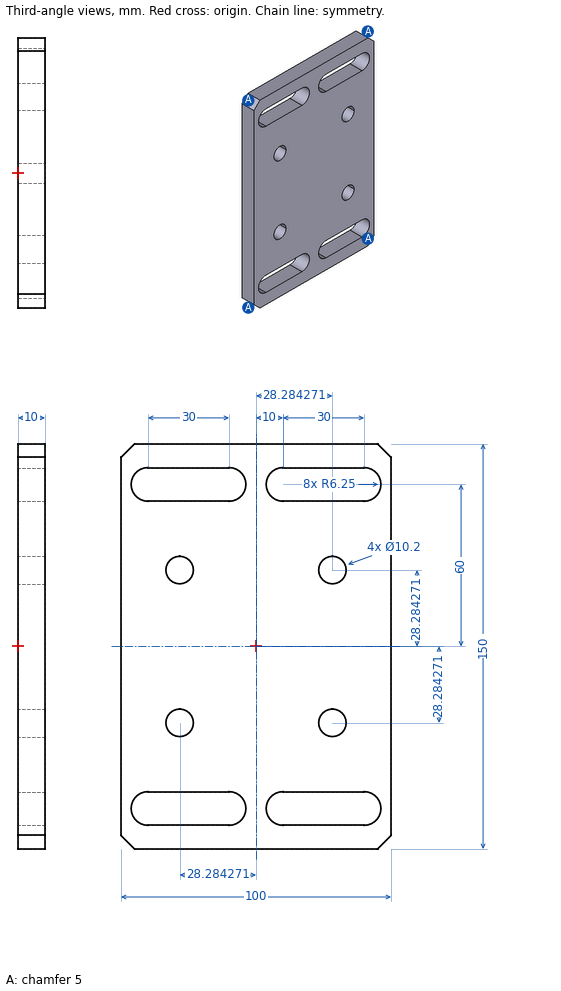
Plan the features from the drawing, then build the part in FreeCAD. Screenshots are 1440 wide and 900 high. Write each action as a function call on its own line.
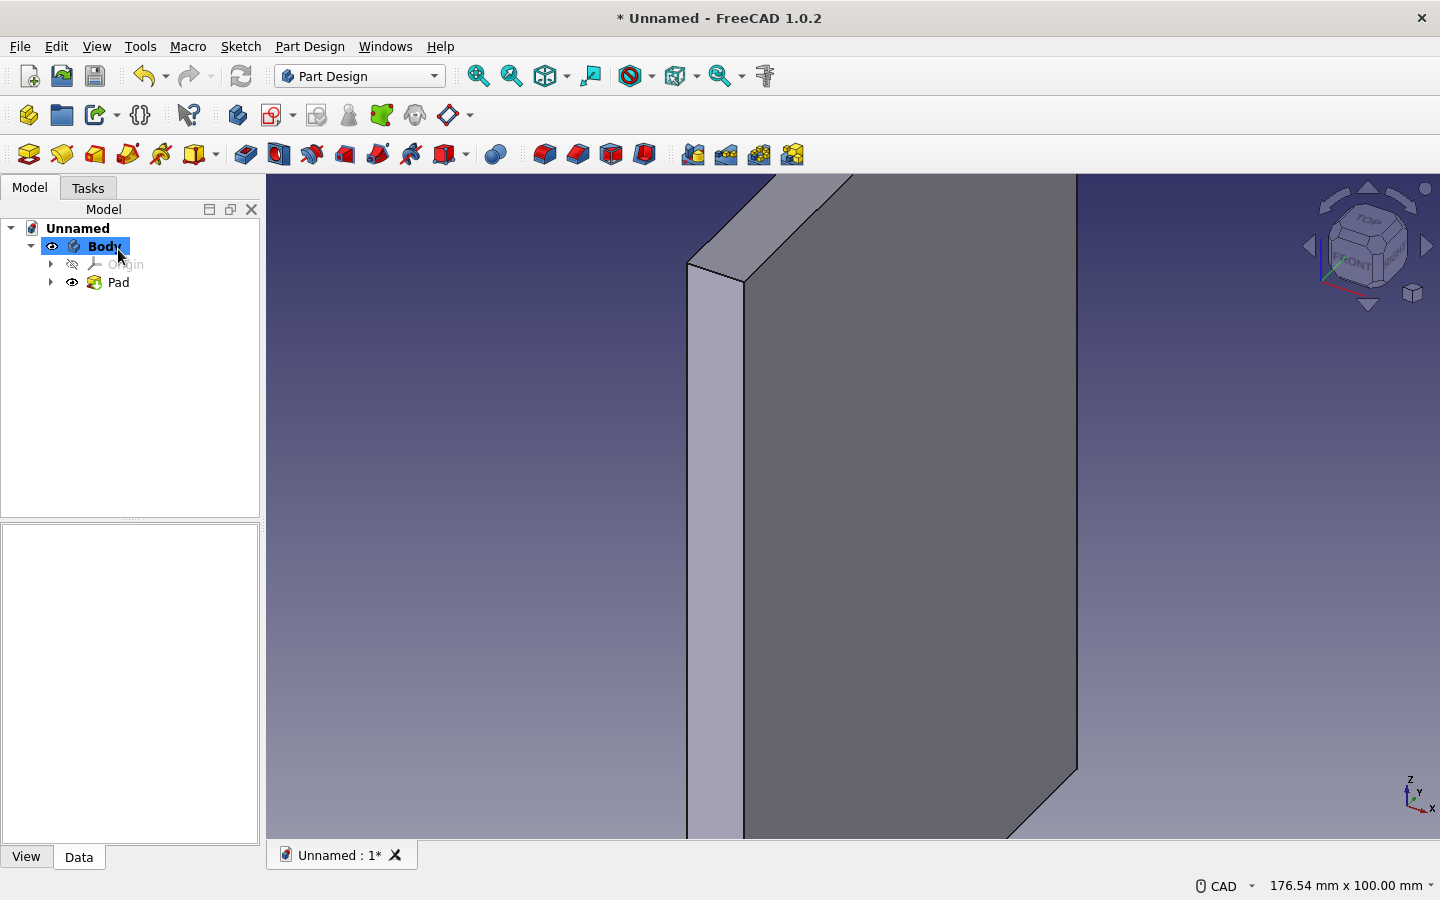
click(479, 76)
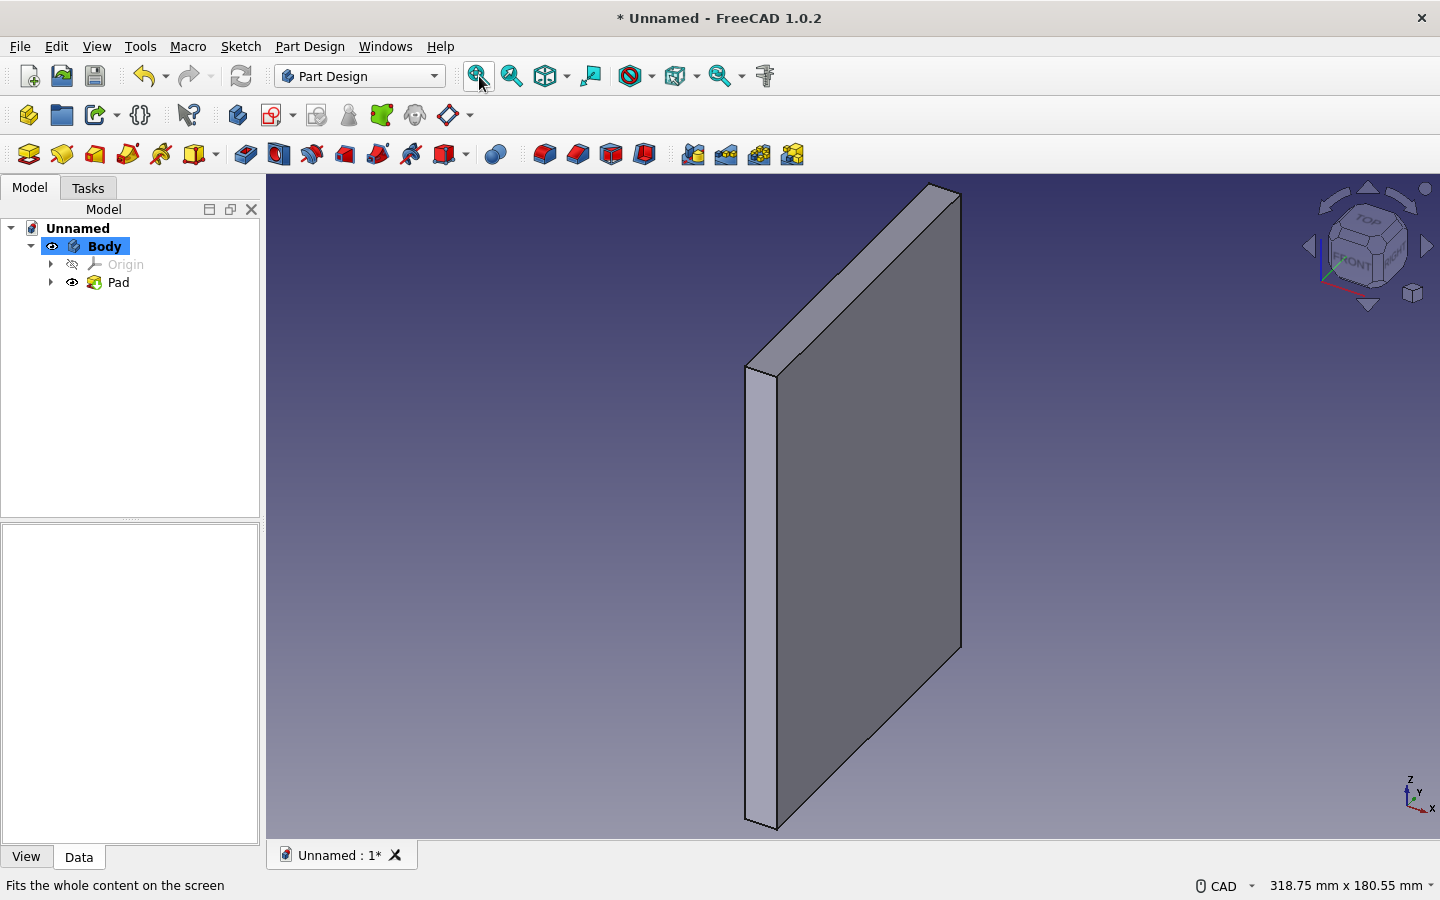
click(869, 575)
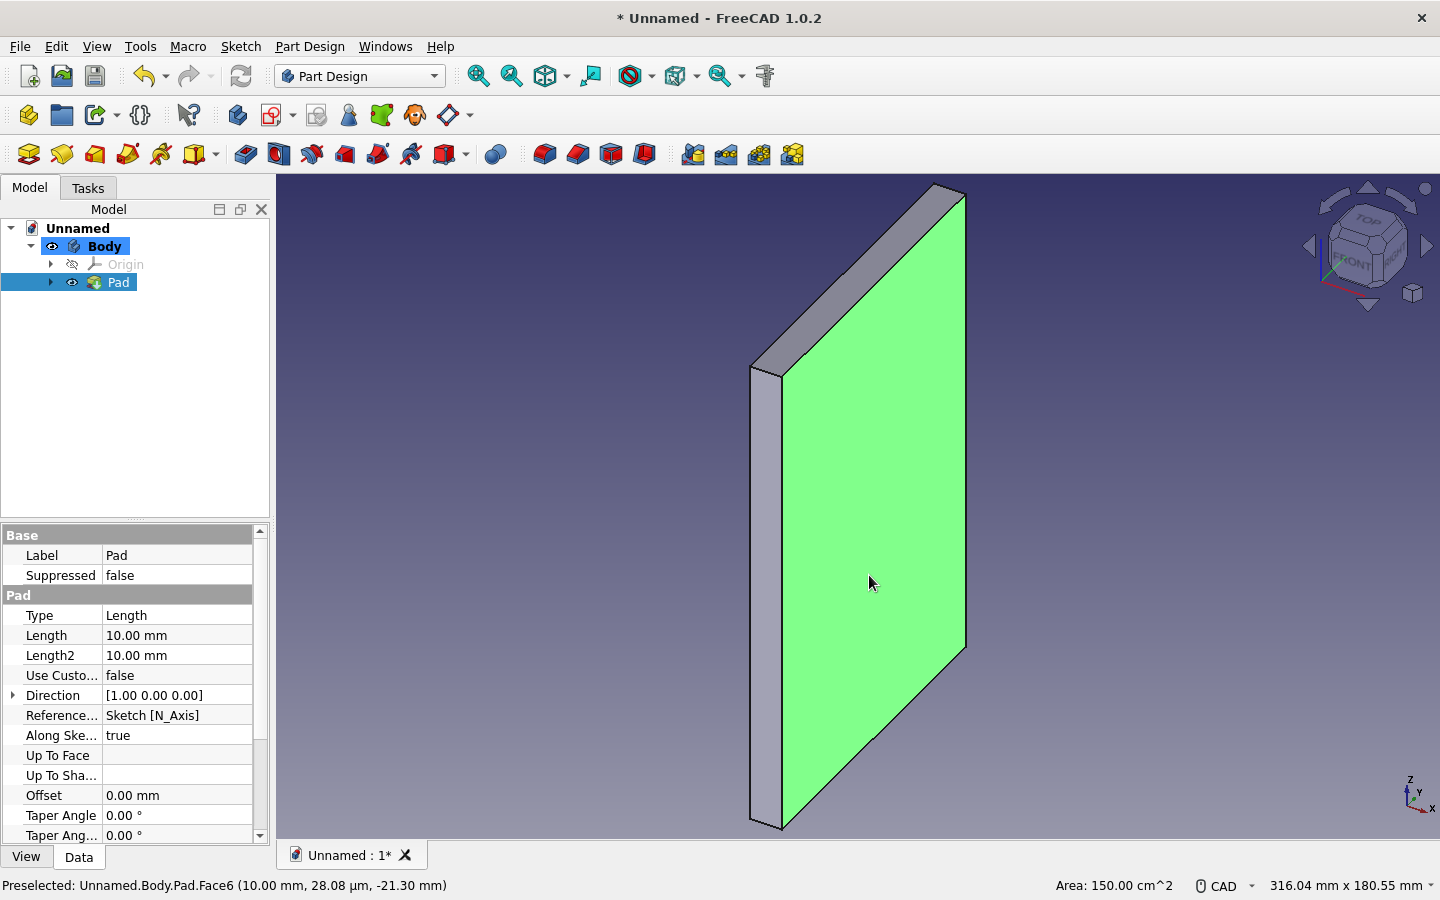
click(270, 116)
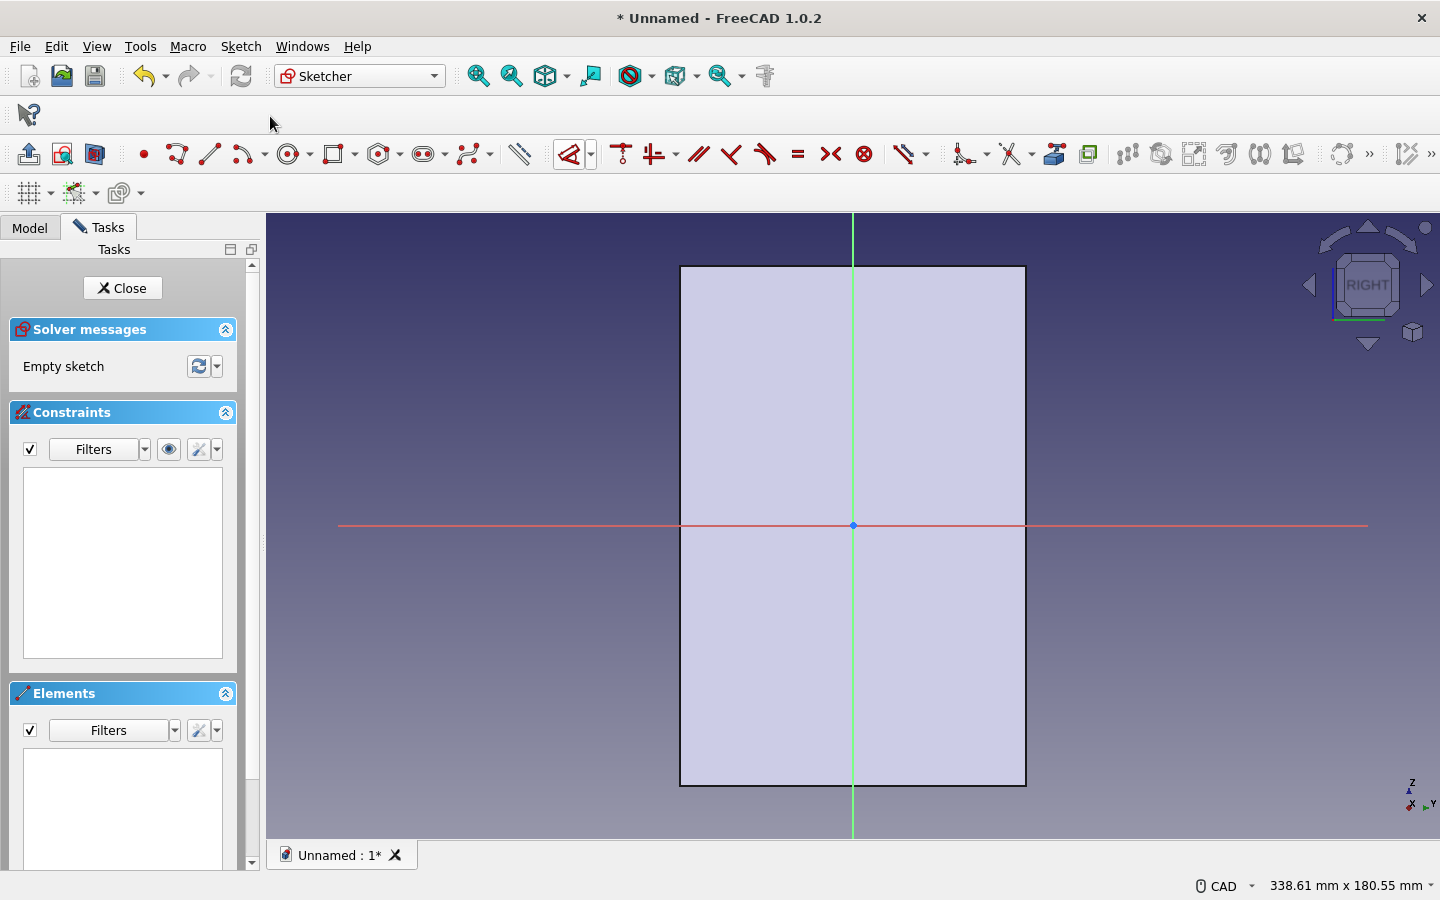
scroll(936, 526, up, 3)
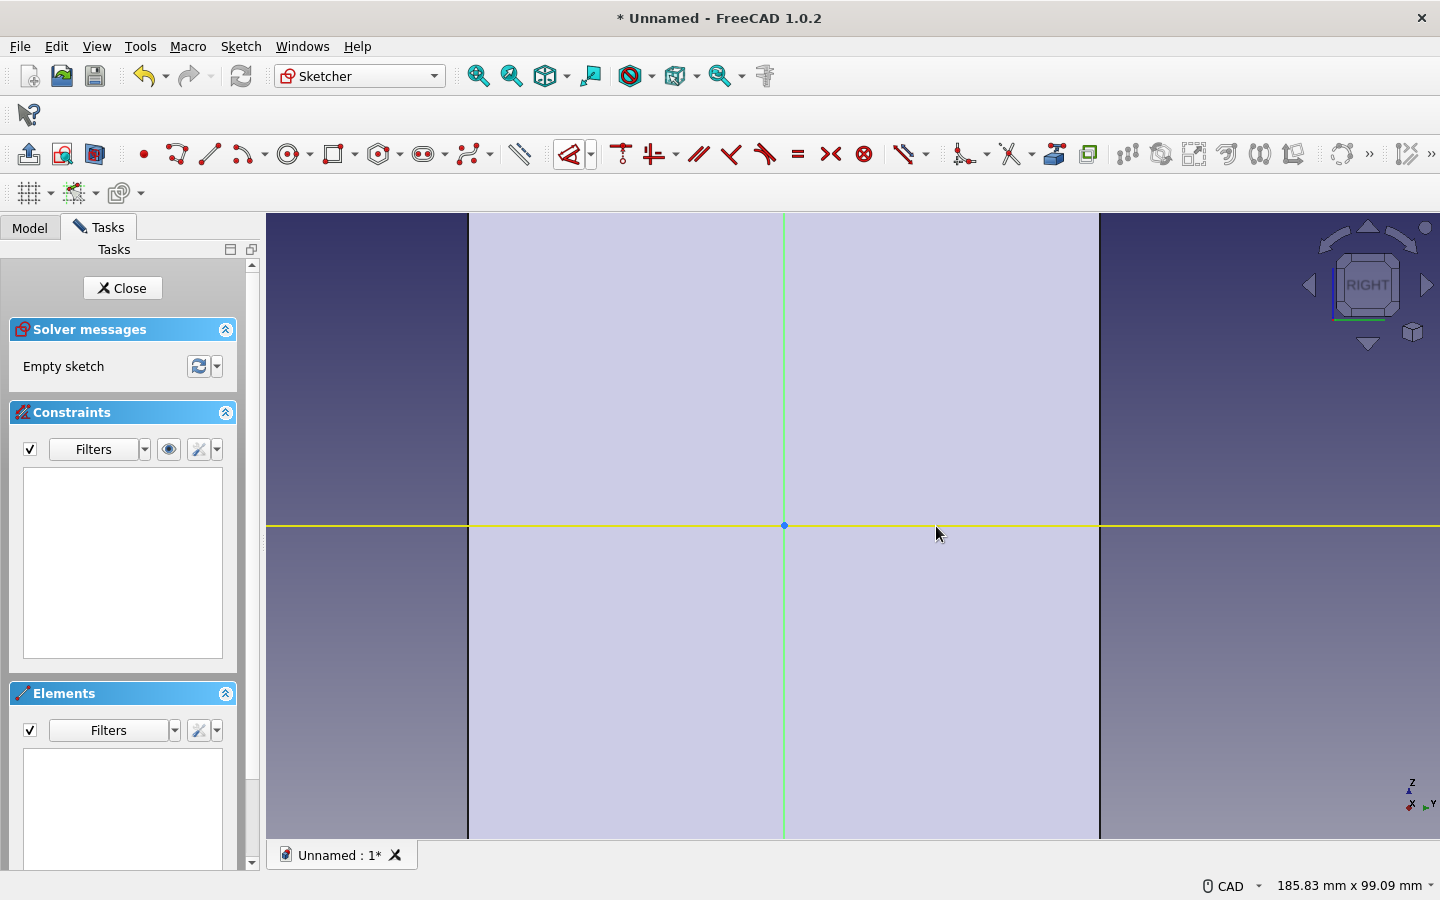
click(288, 154)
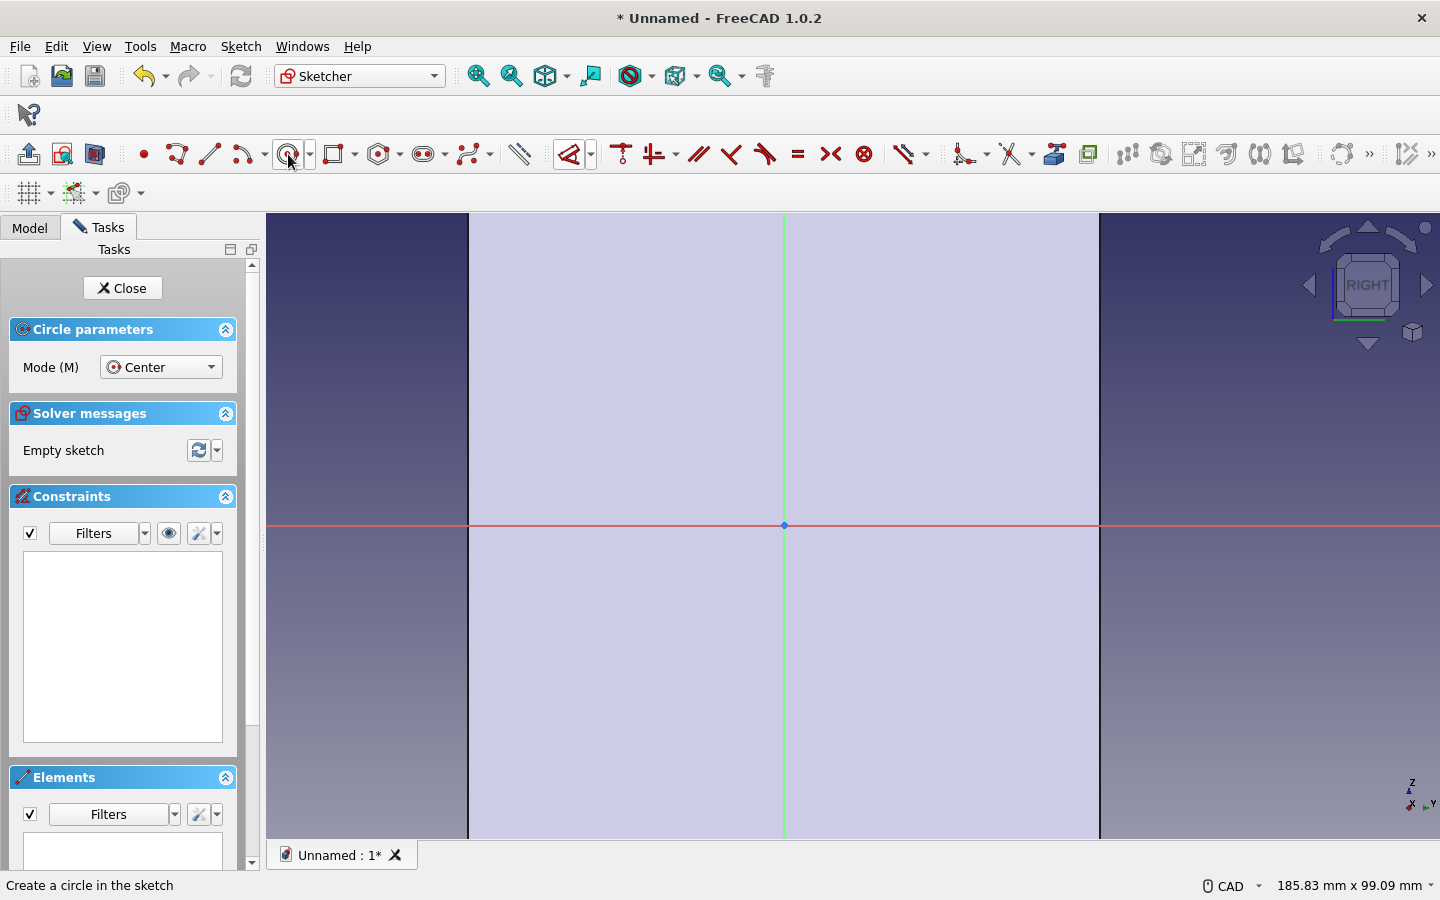
click(963, 347)
click(986, 324)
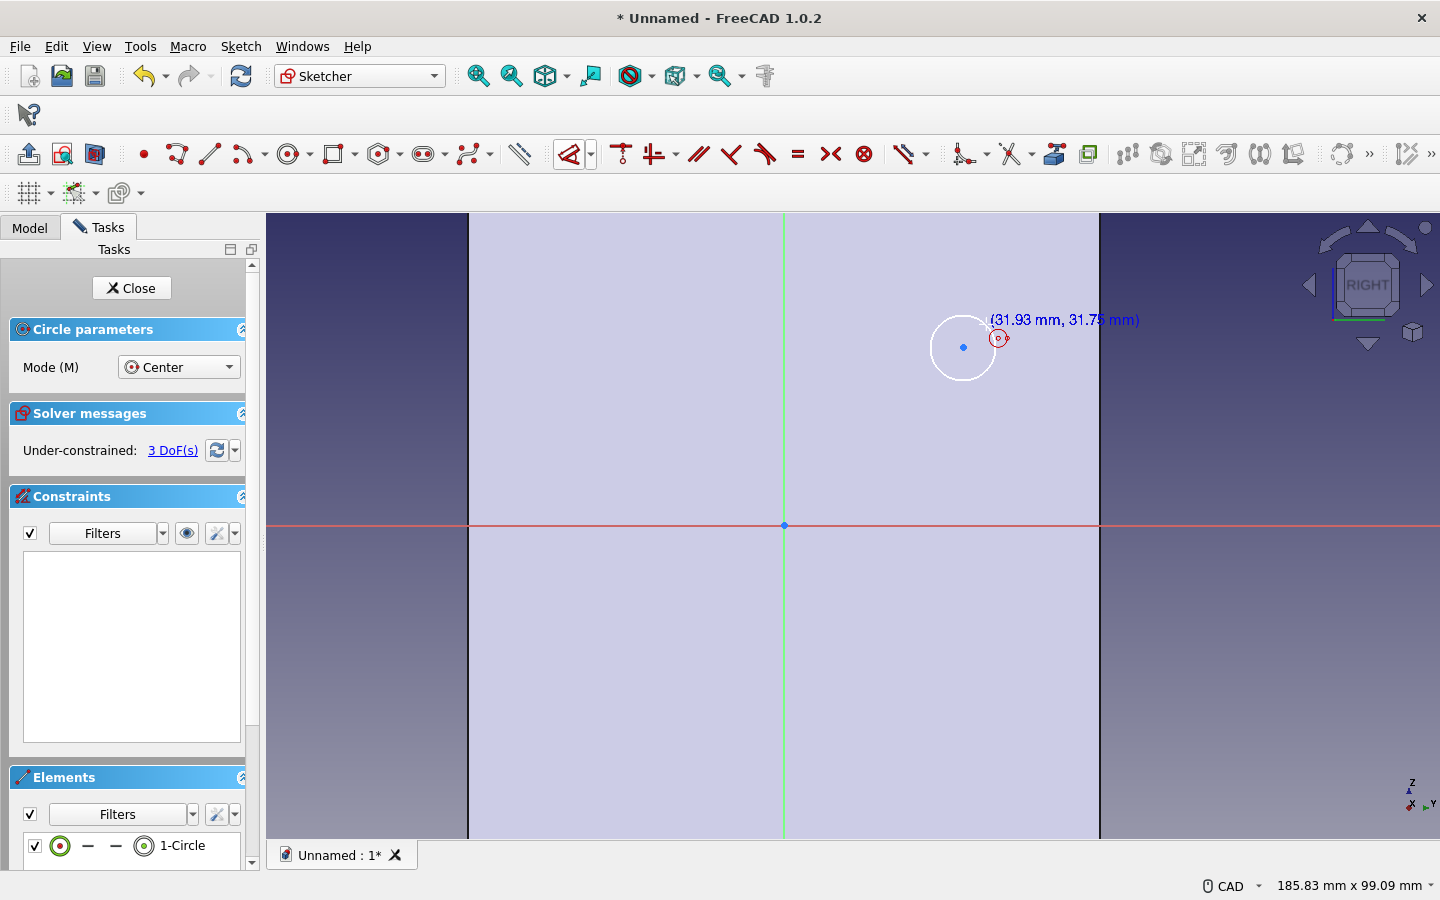
click(963, 704)
click(986, 681)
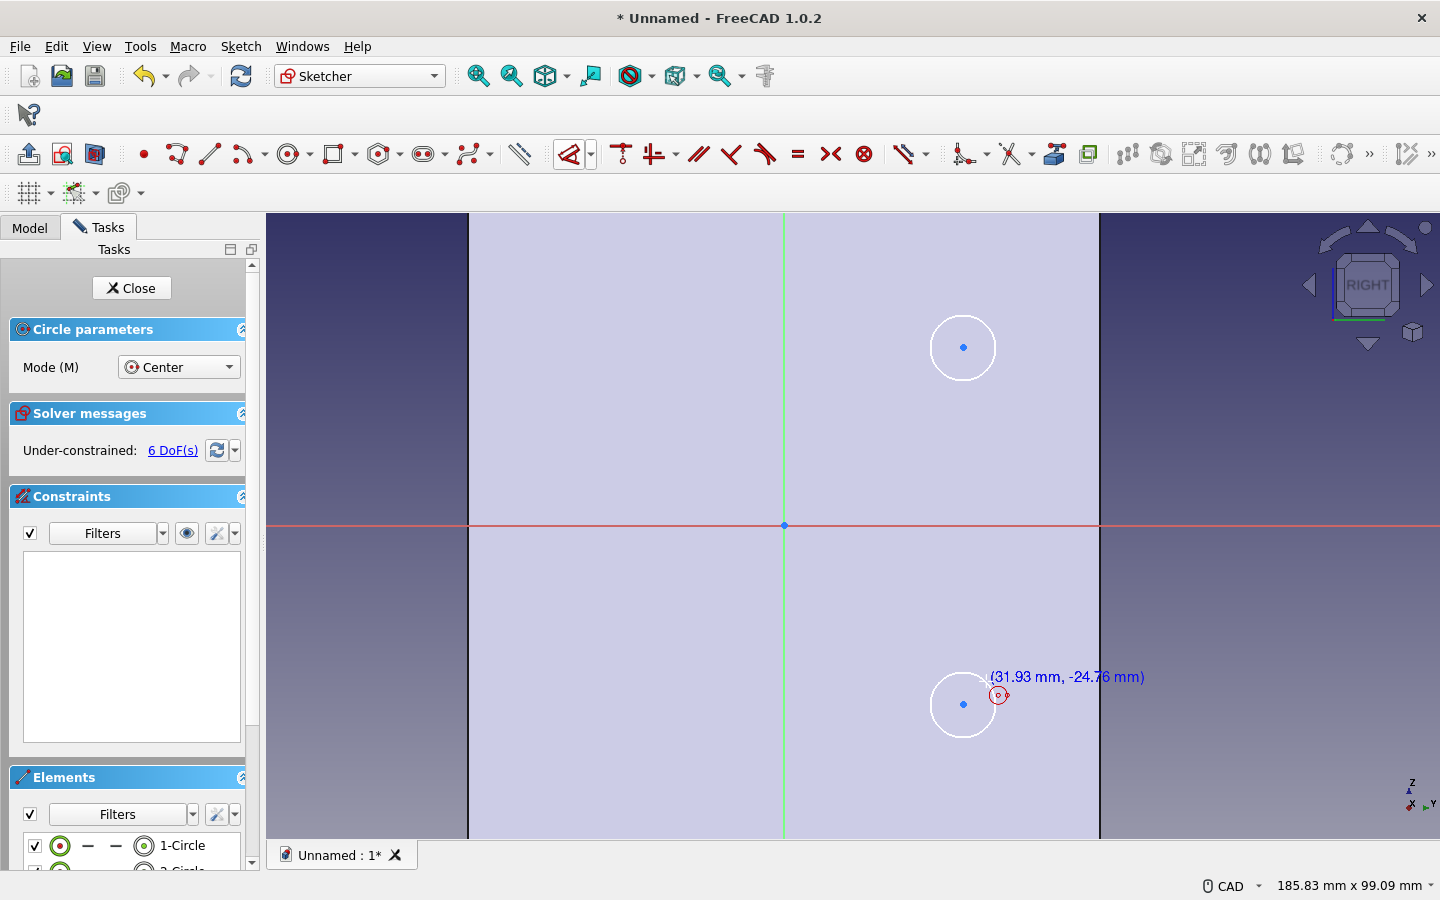
click(606, 704)
click(628, 681)